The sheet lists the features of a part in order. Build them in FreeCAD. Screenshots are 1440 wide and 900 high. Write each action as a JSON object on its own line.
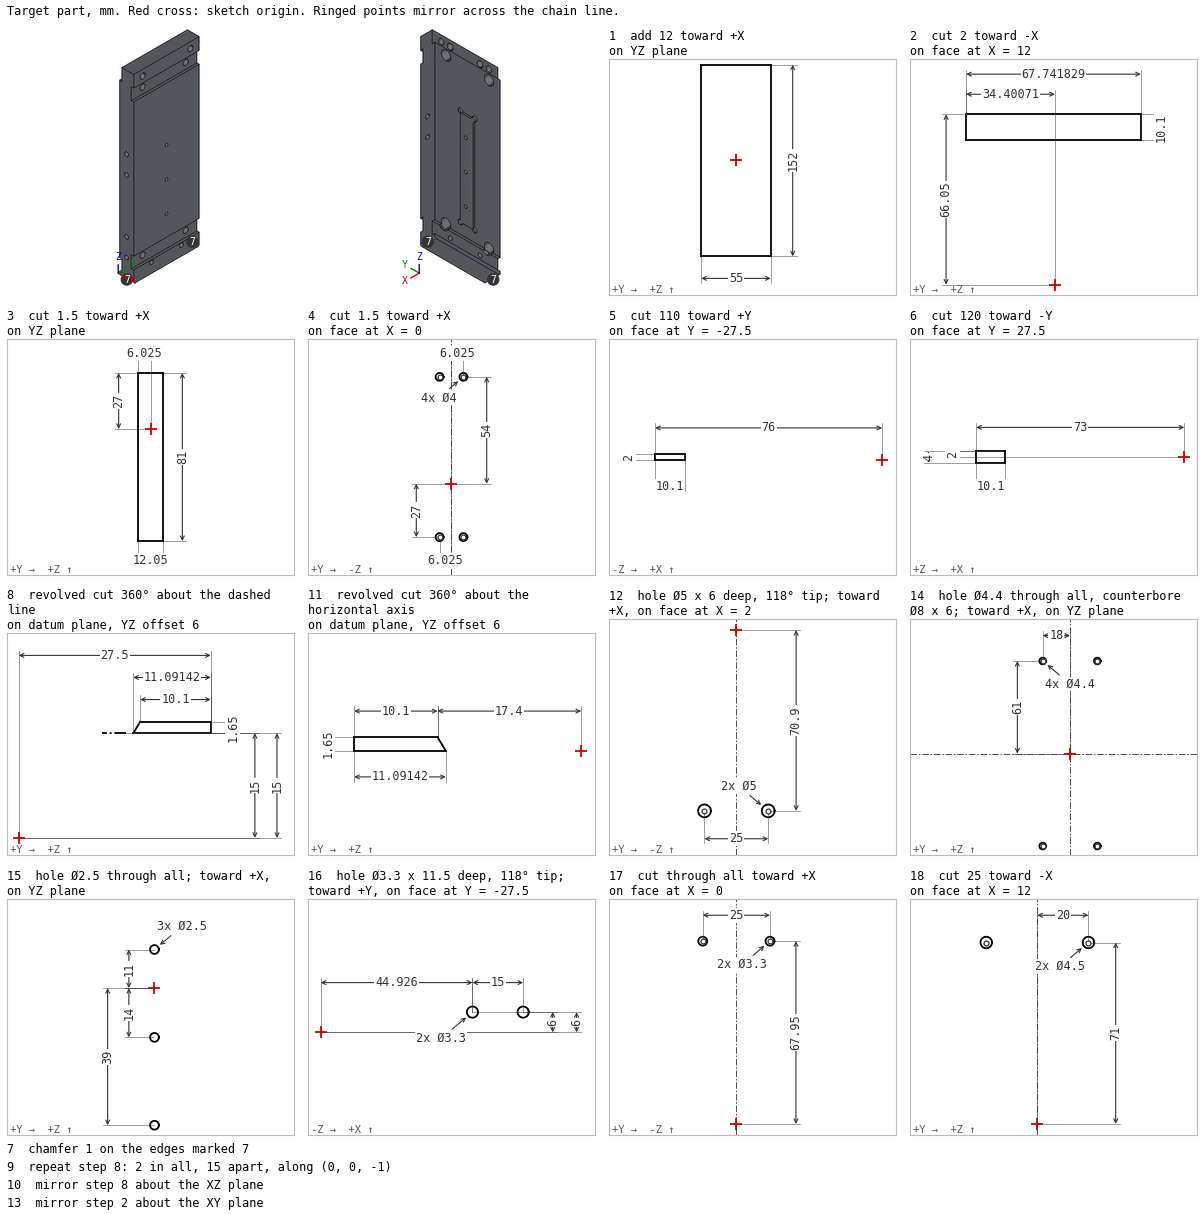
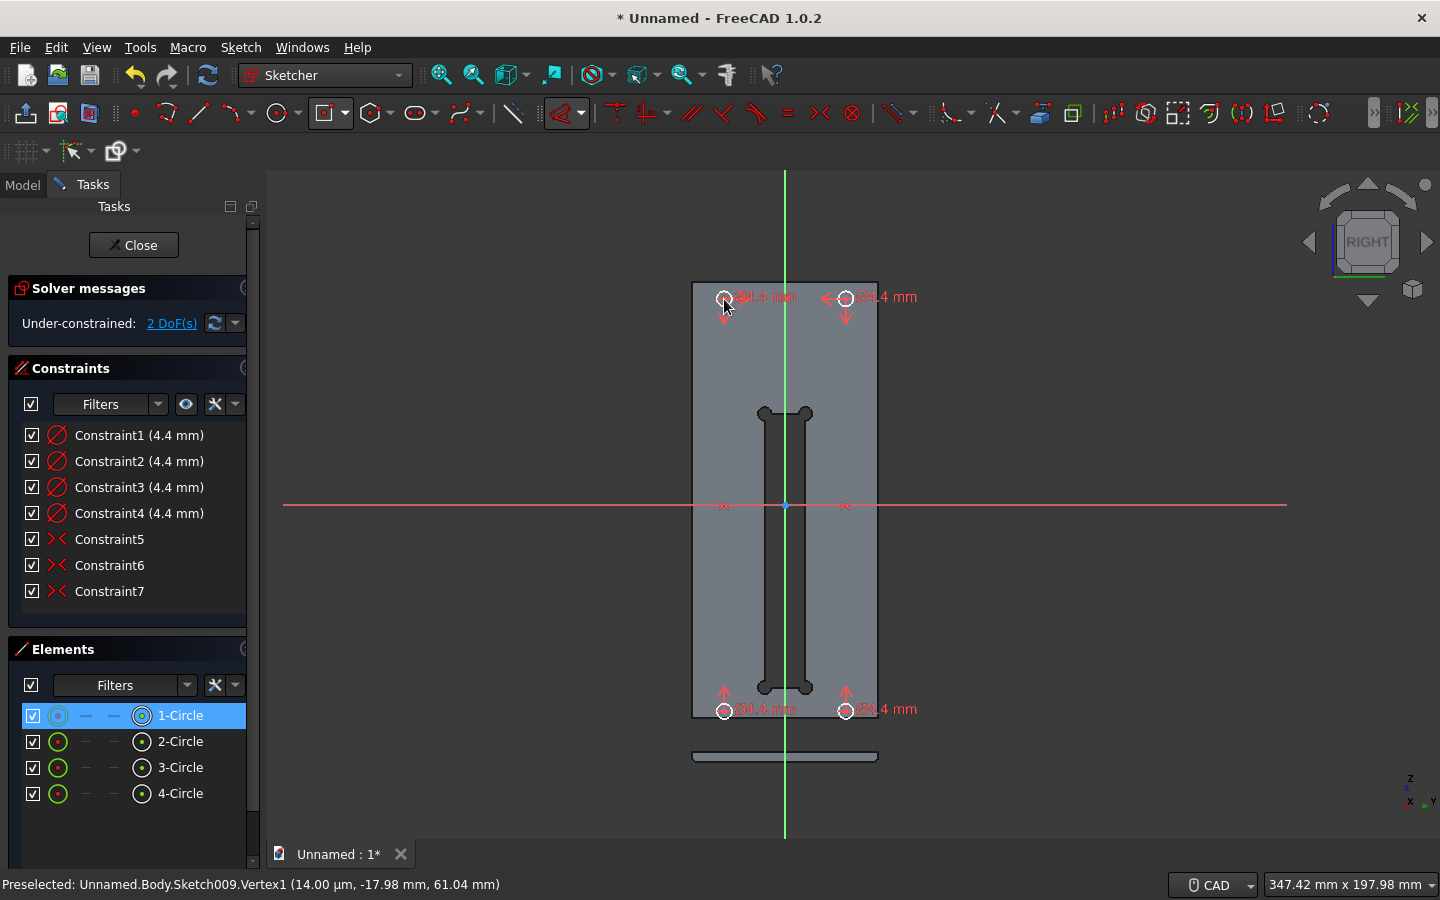
{"action": "key", "text": "l"}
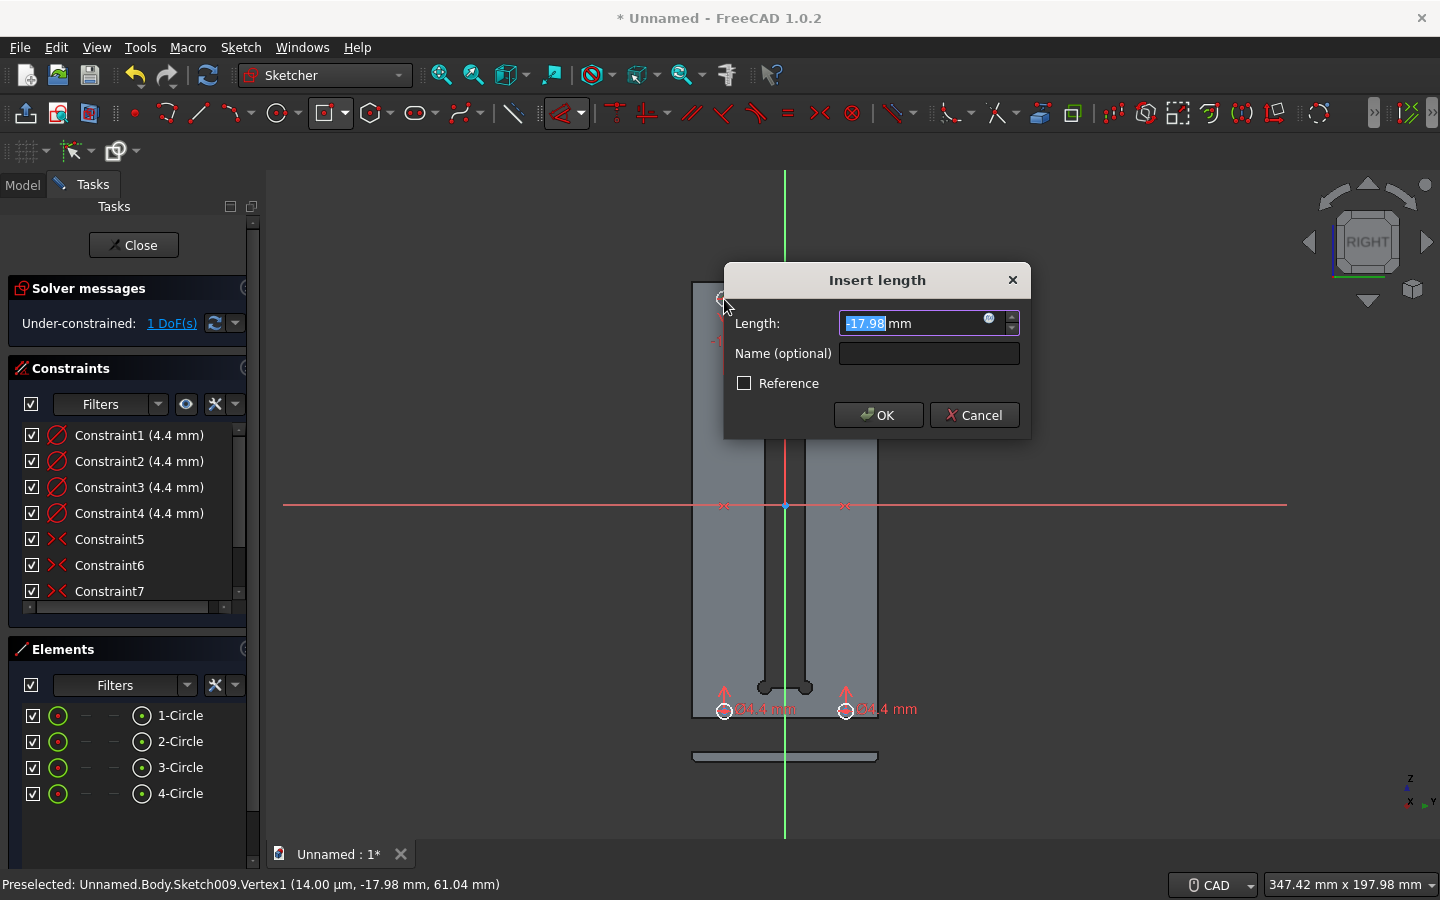
{"action": "type", "text": "-18"}
{"action": "key", "text": "Return"}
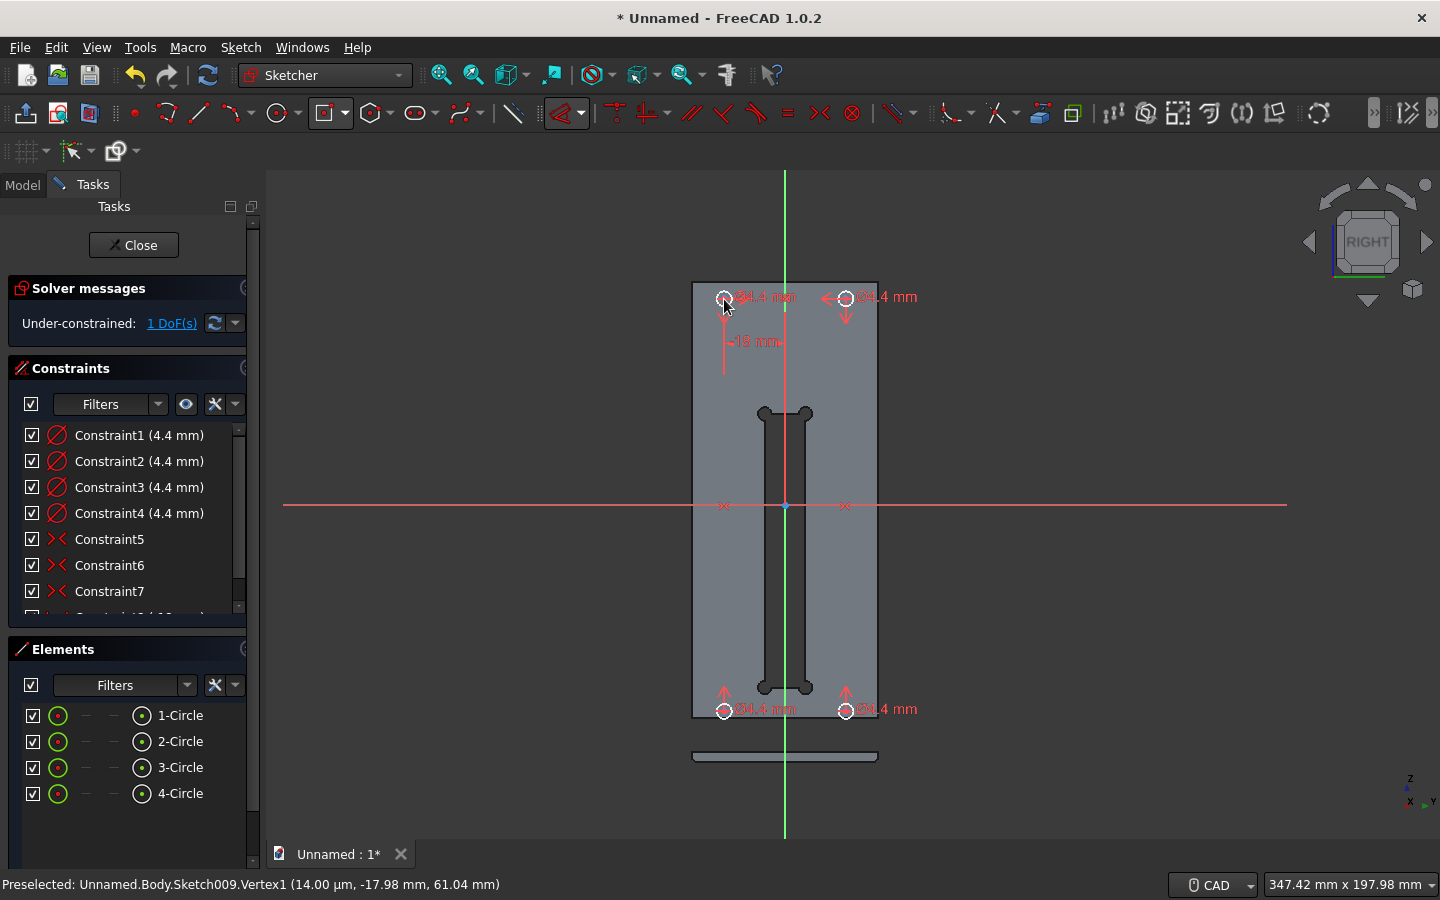
{"action": "left_click", "coordinate": [724, 299]}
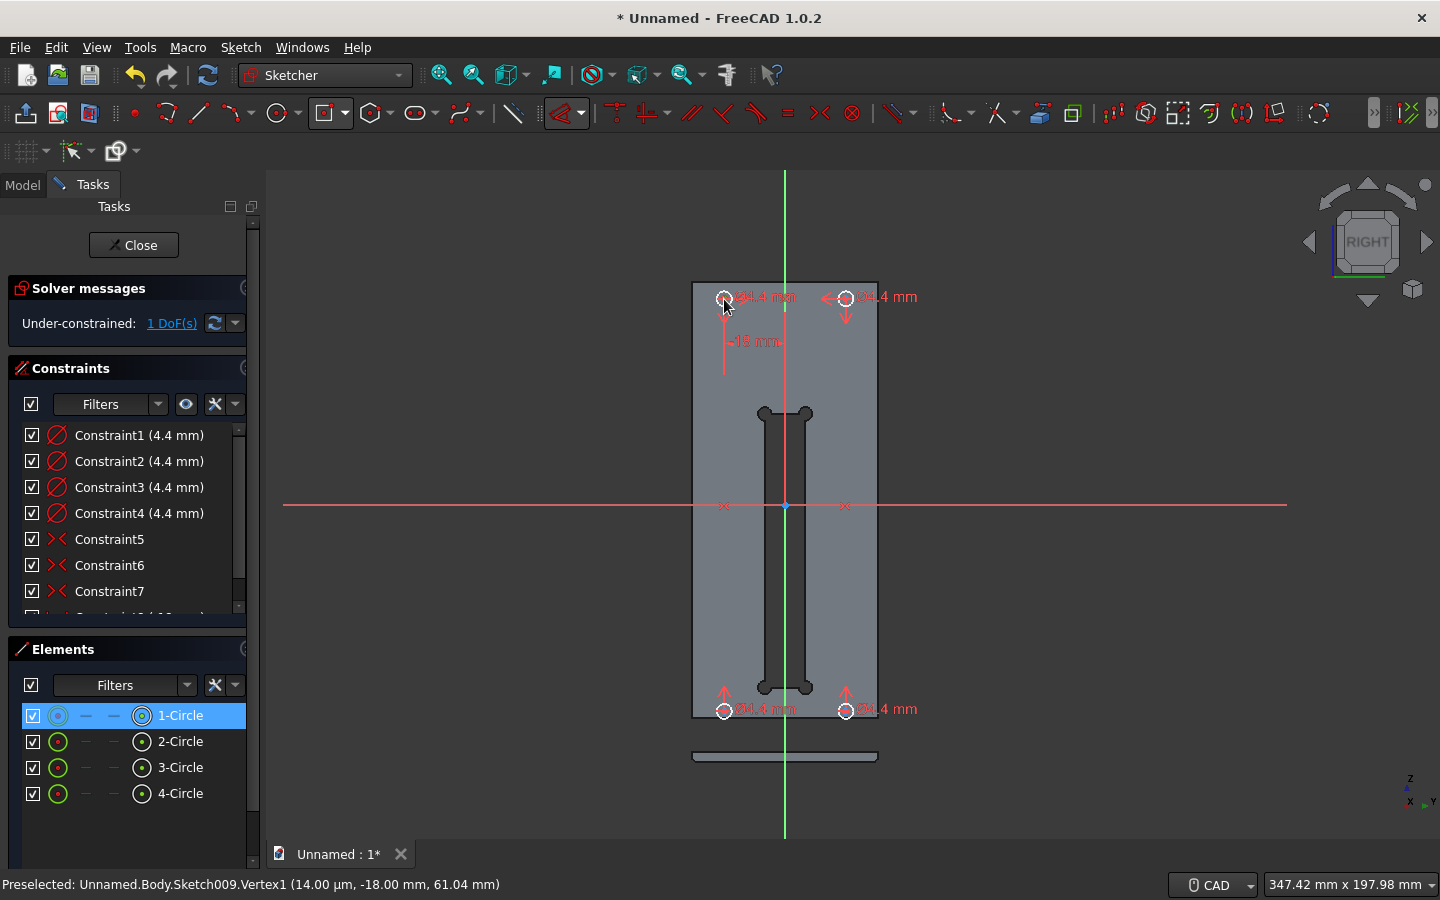
{"action": "left_click", "coordinate": [584, 114]}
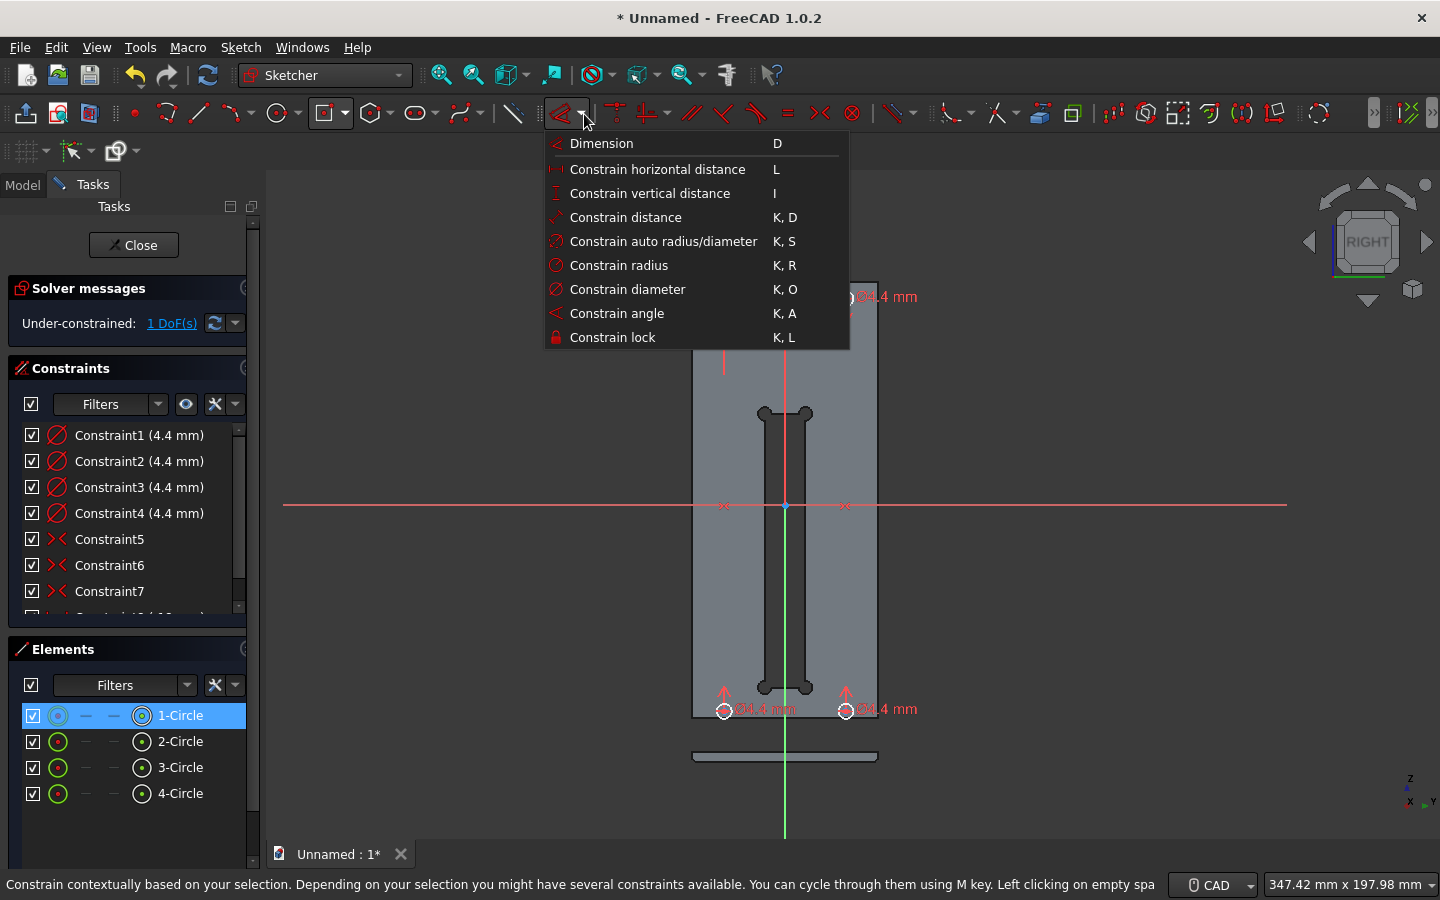
{"action": "left_click", "coordinate": [697, 193]}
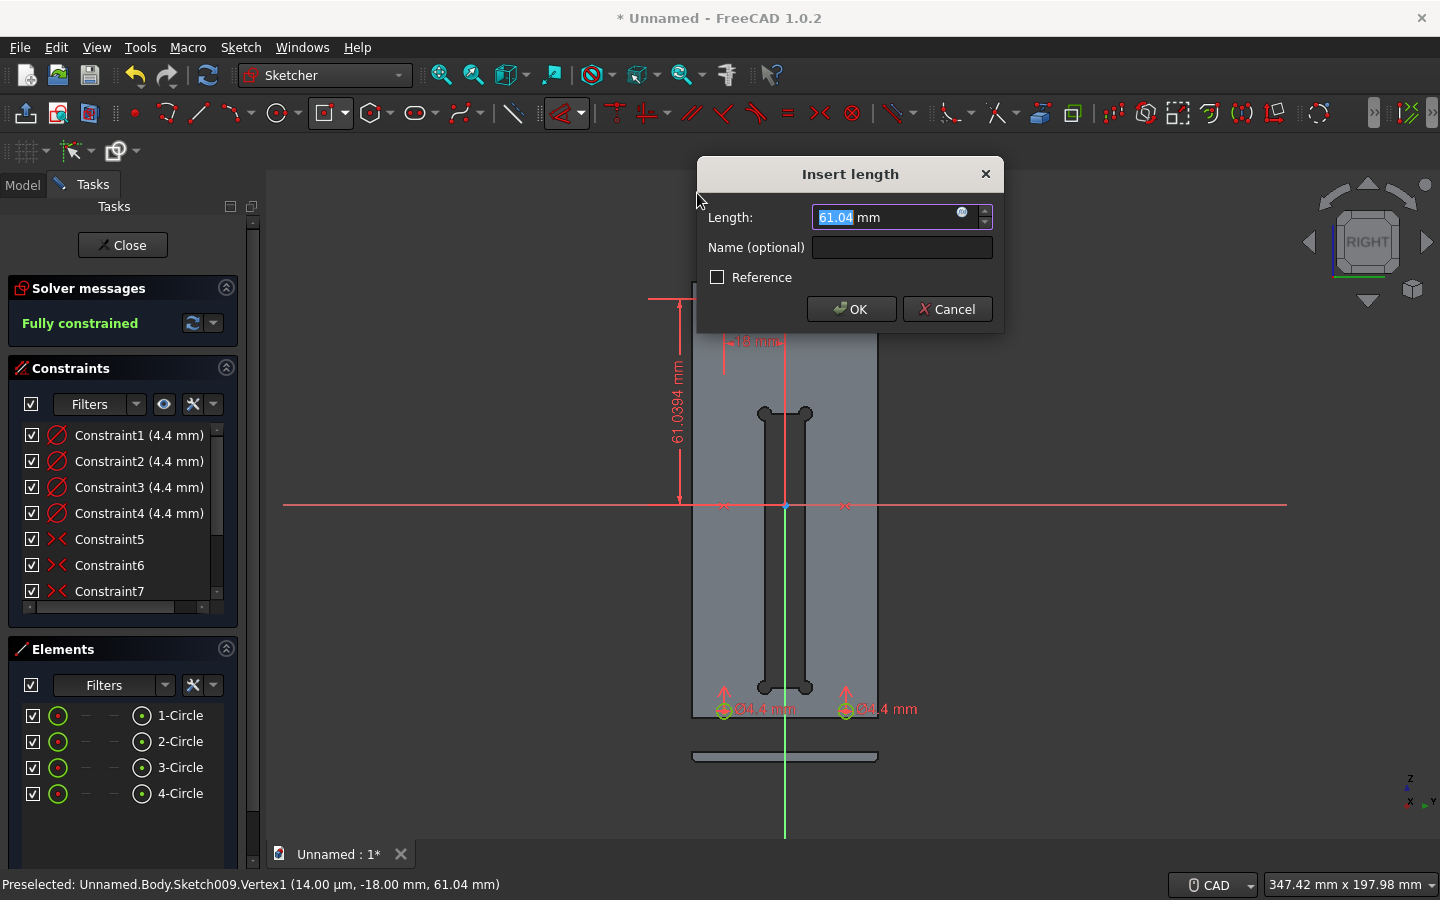
{"action": "type", "text": "61"}
{"action": "key", "text": "Return"}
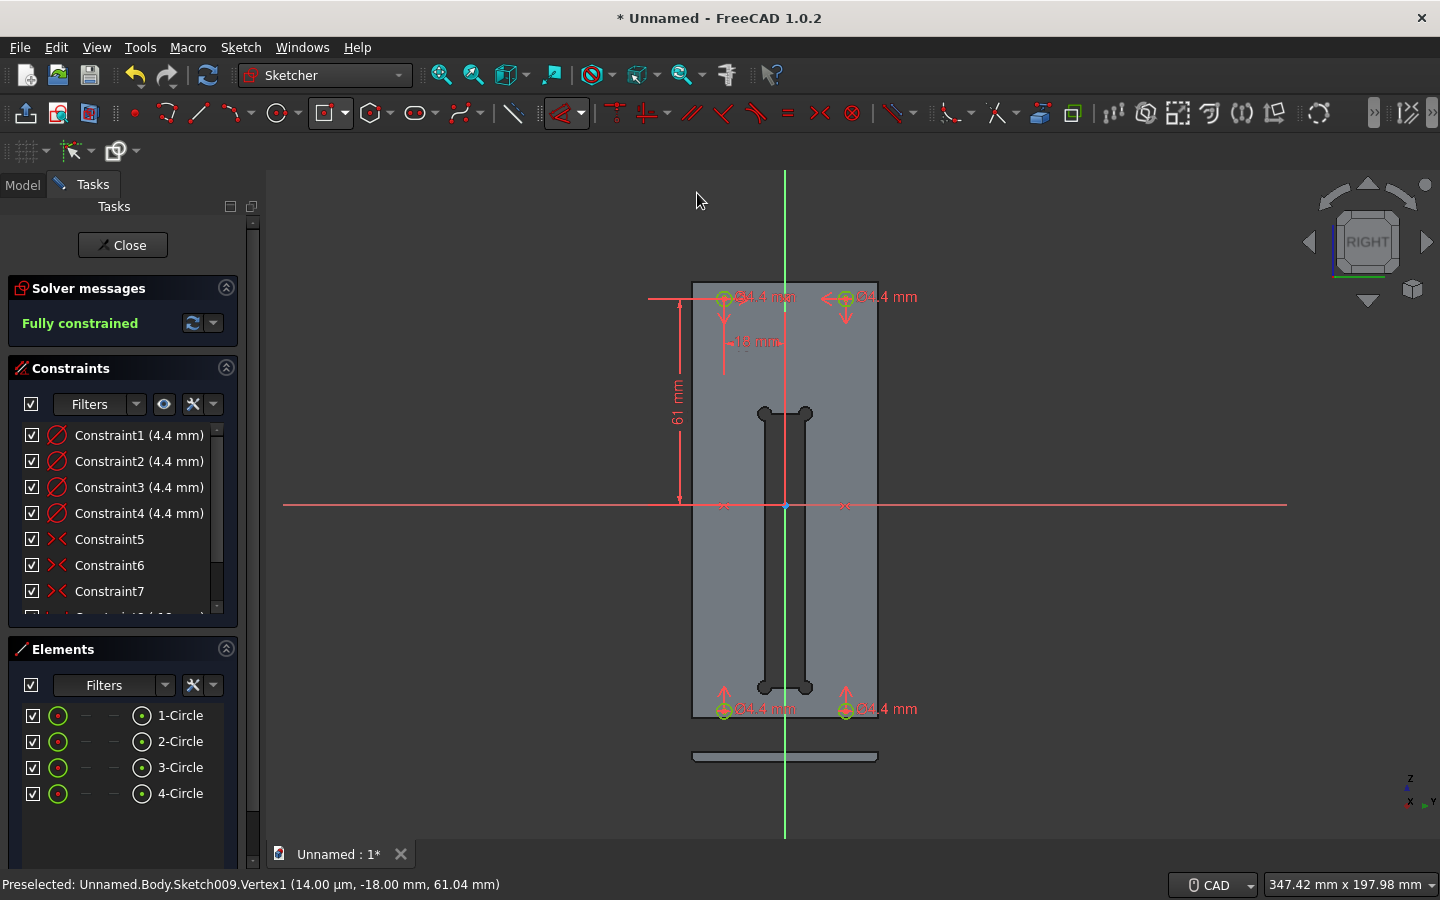
{"action": "left_click", "coordinate": [123, 245]}